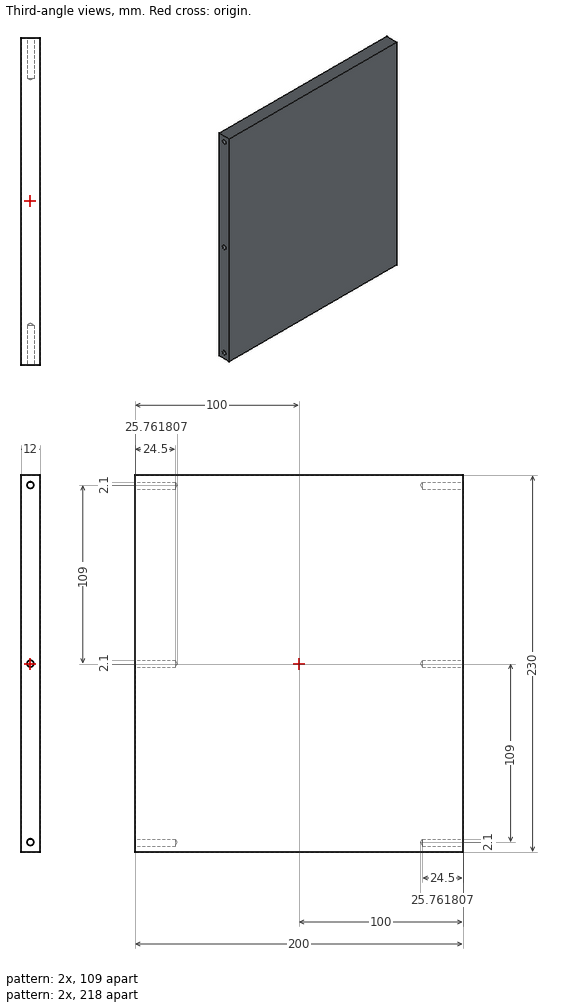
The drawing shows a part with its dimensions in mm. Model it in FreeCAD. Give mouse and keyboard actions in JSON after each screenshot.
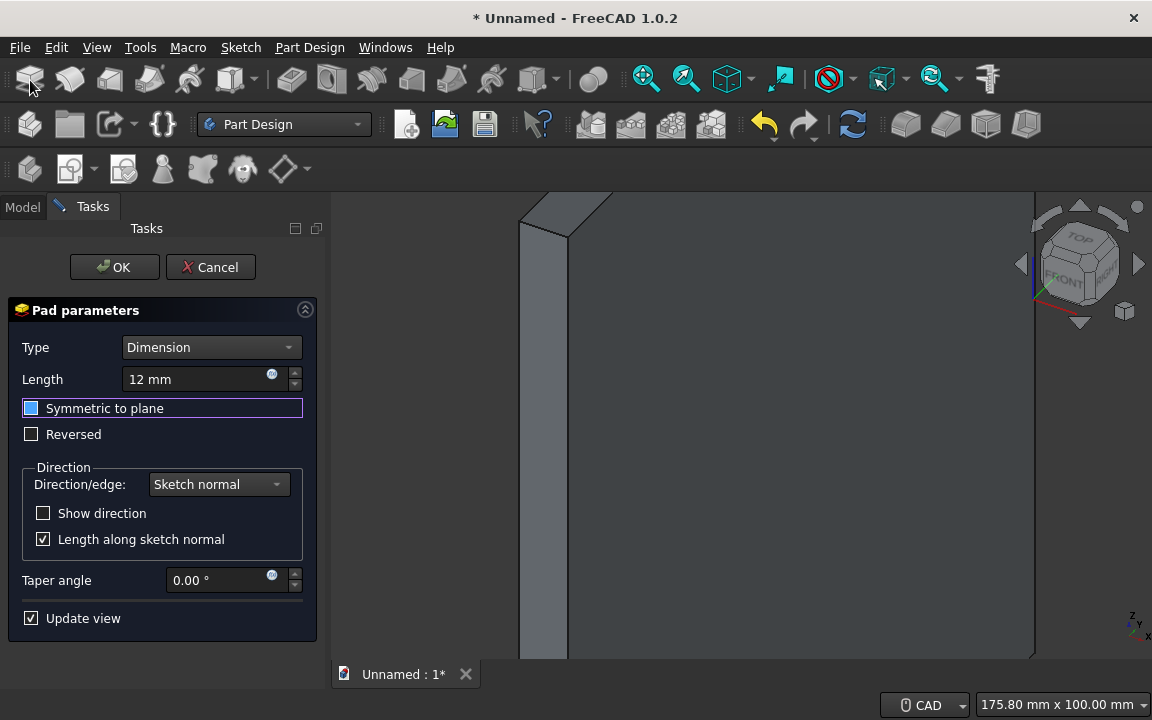
{"action": "left_click", "coordinate": [30, 408]}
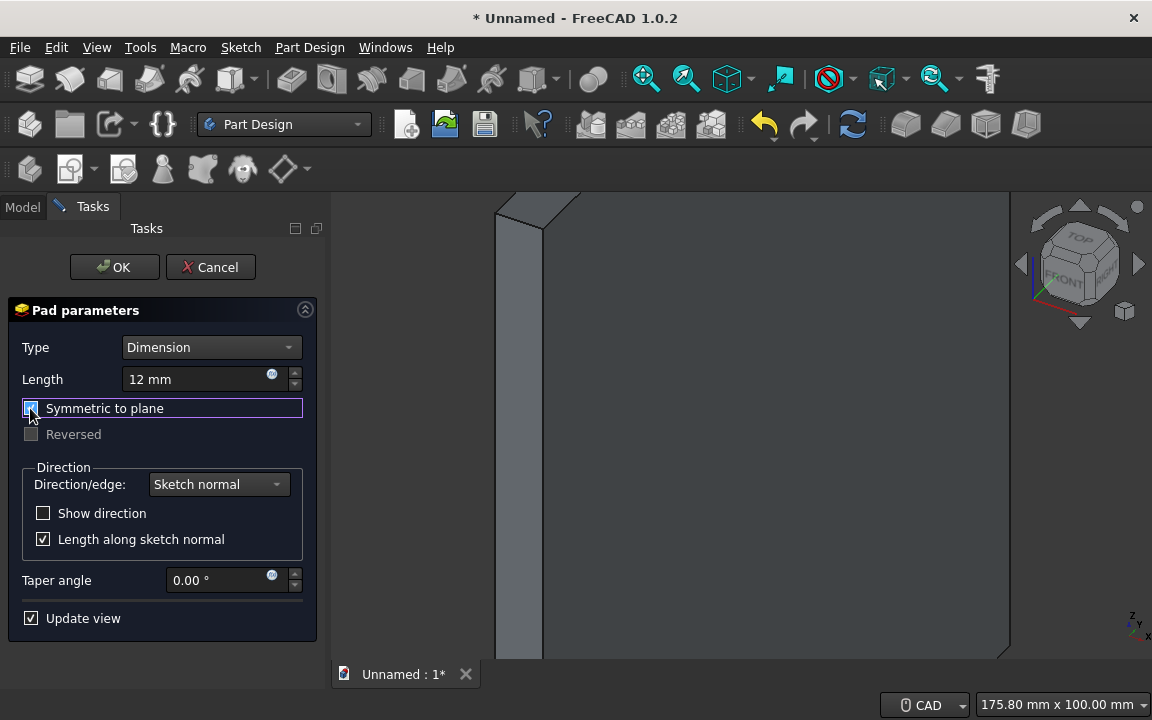
{"action": "left_click", "coordinate": [115, 267]}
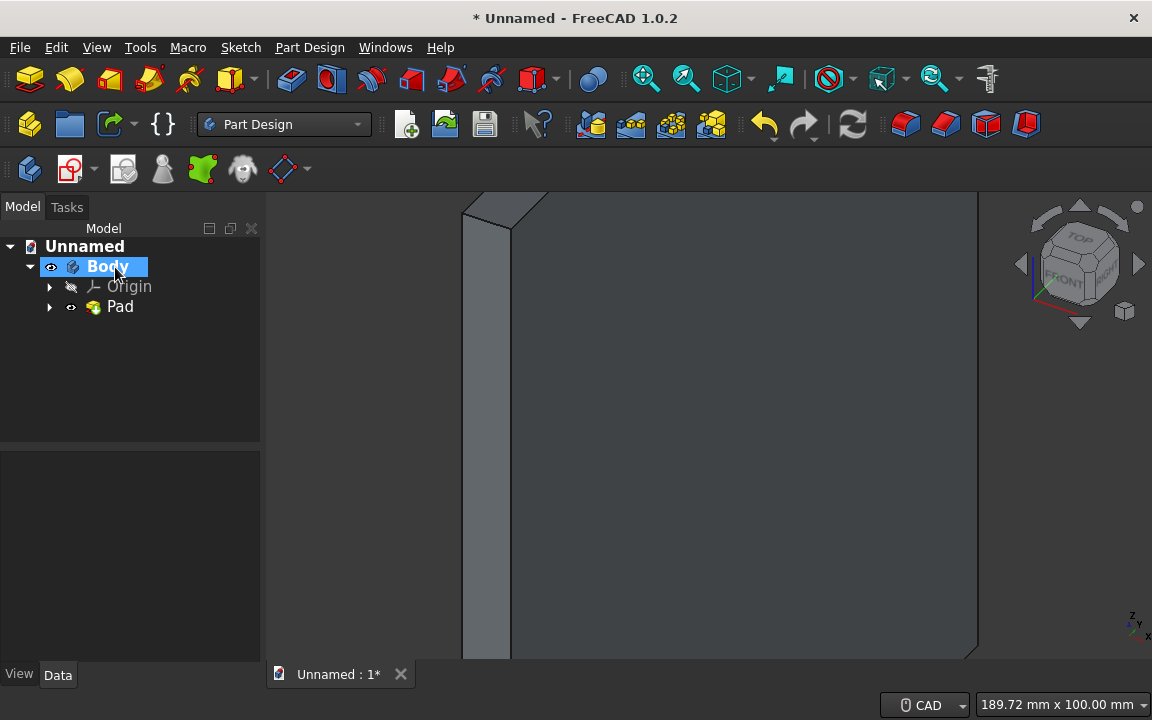
{"action": "left_click", "coordinate": [648, 80]}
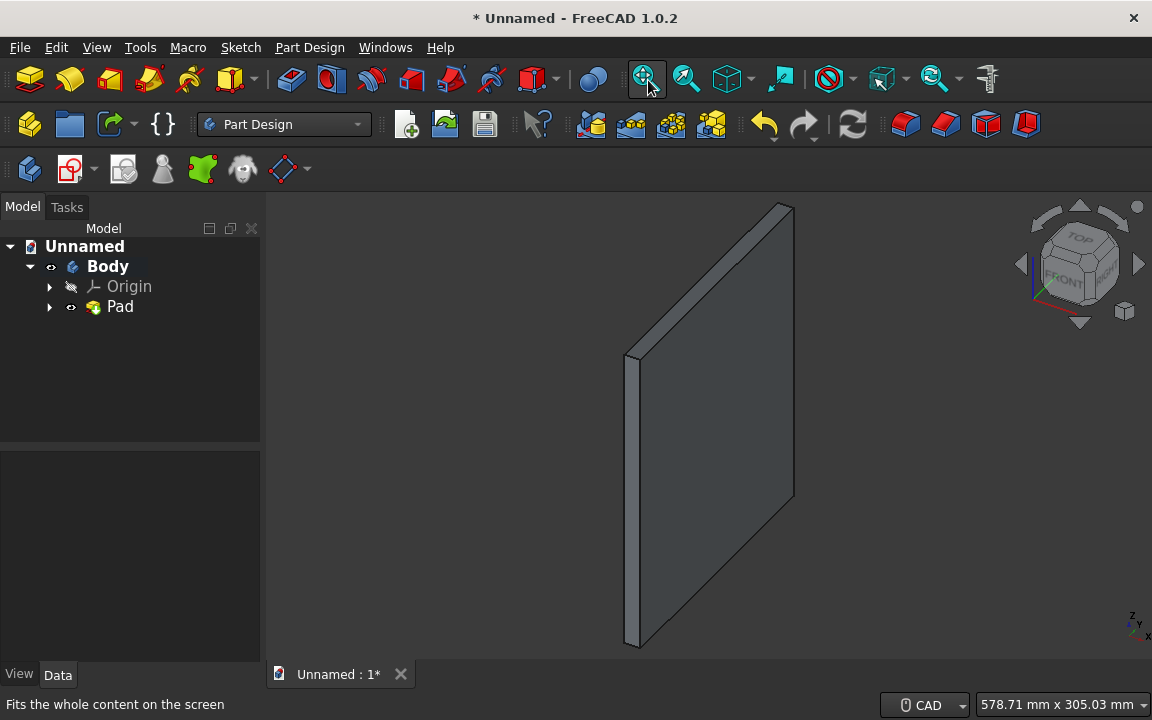
{"action": "left_click", "coordinate": [70, 170]}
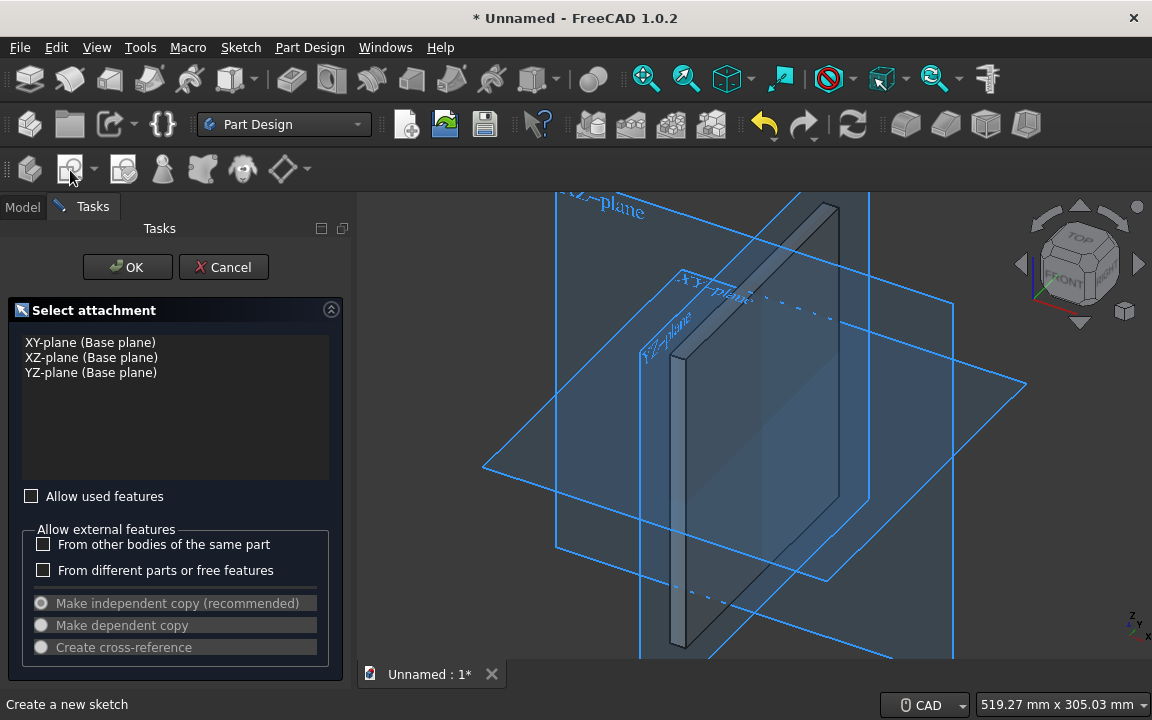
{"action": "left_click", "coordinate": [82, 372]}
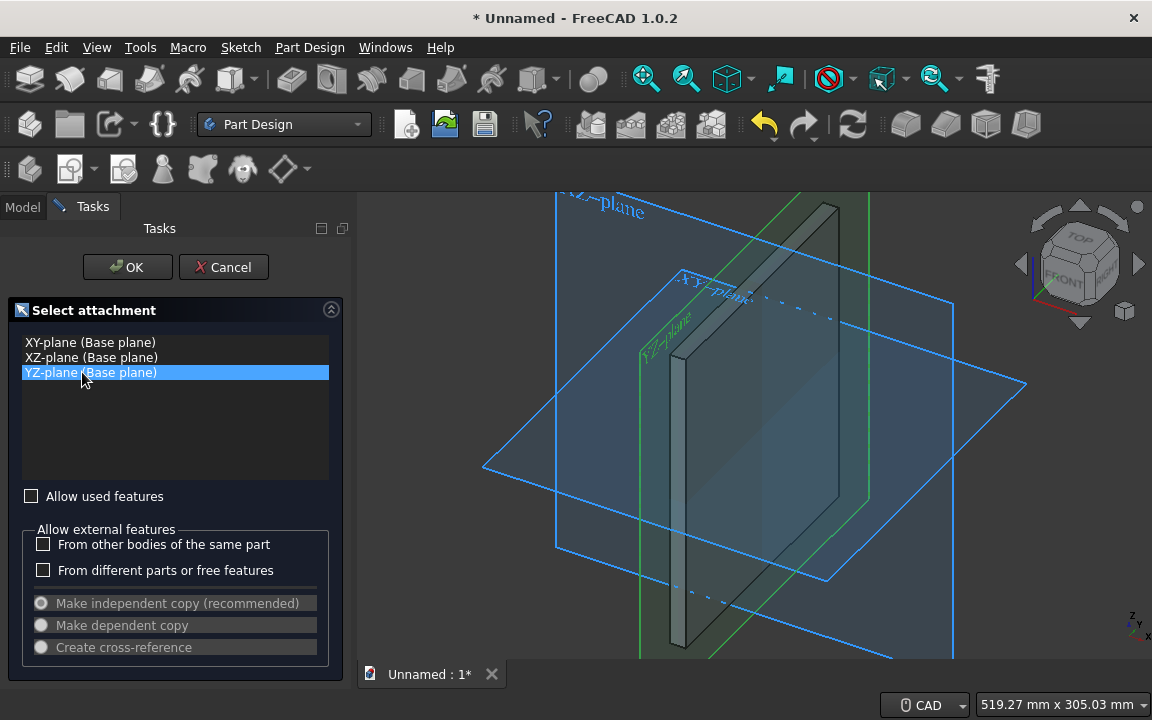
{"action": "left_click", "coordinate": [128, 267]}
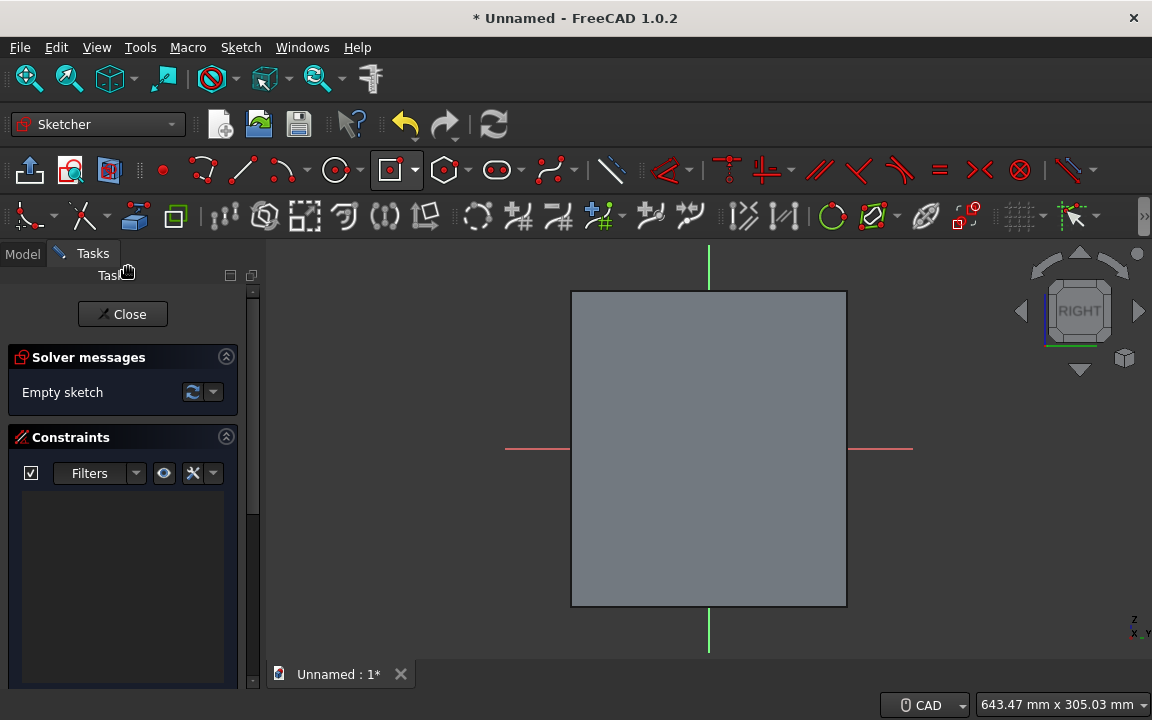
{"action": "left_click", "coordinate": [110, 170]}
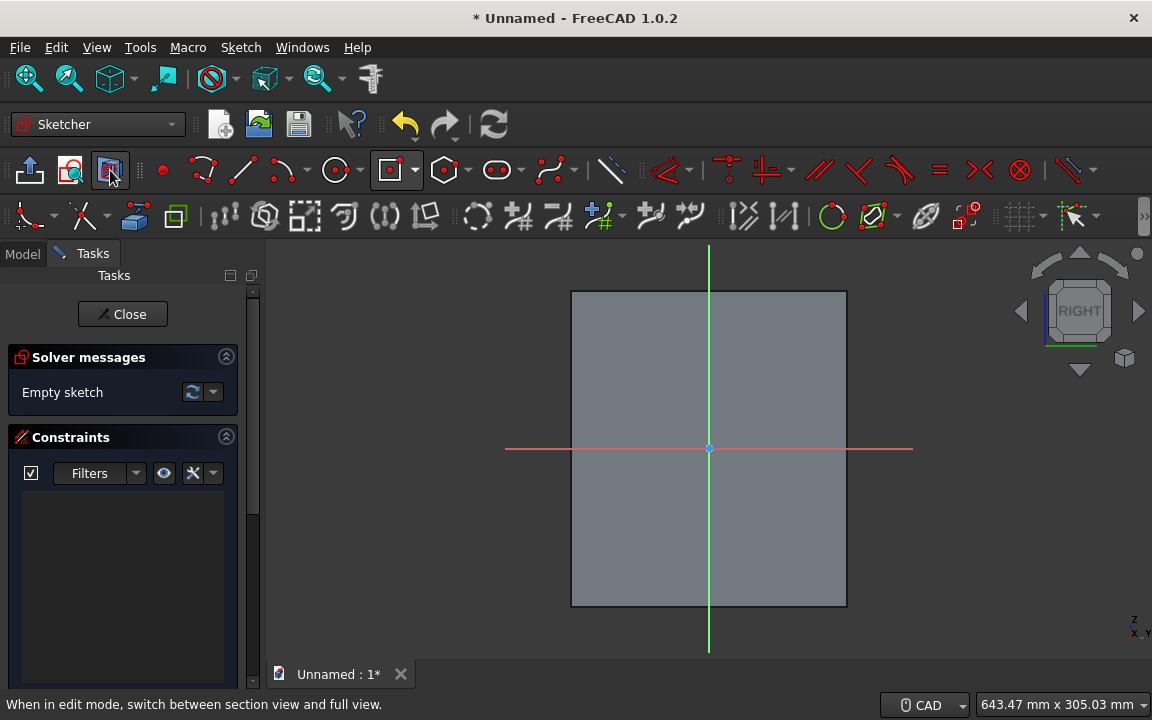
{"action": "scroll", "coordinate": [844, 616], "scroll_direction": "up", "scroll_amount": 11}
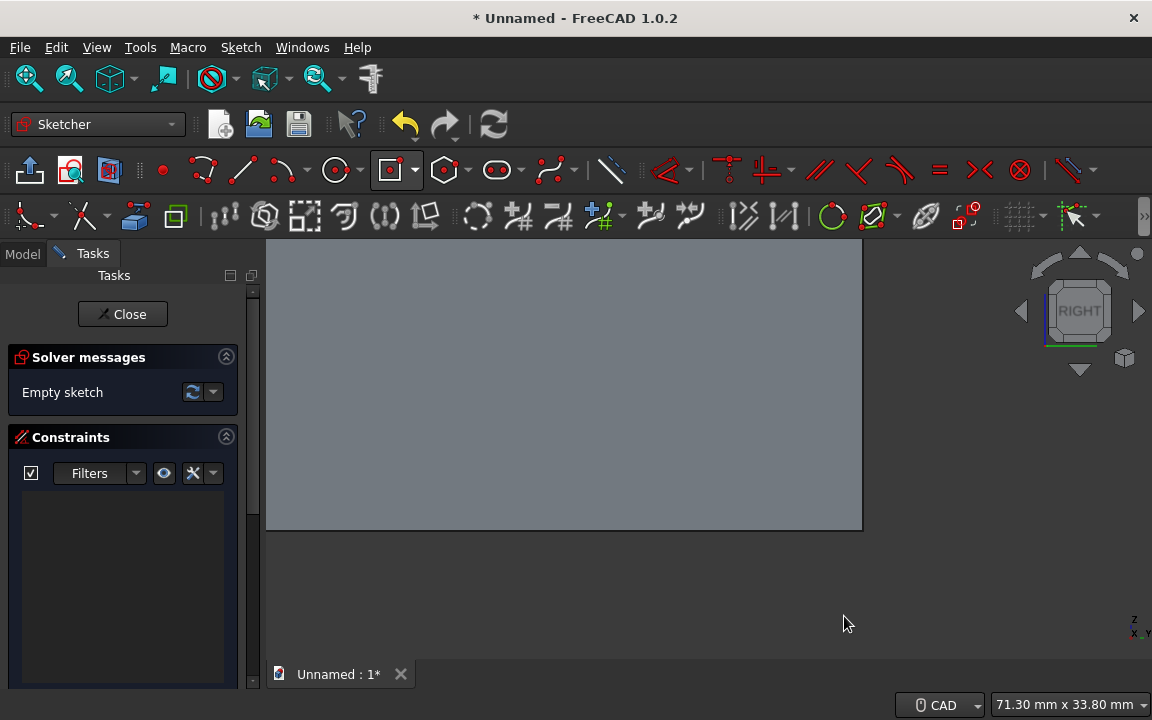
{"action": "left_click", "coordinate": [204, 170]}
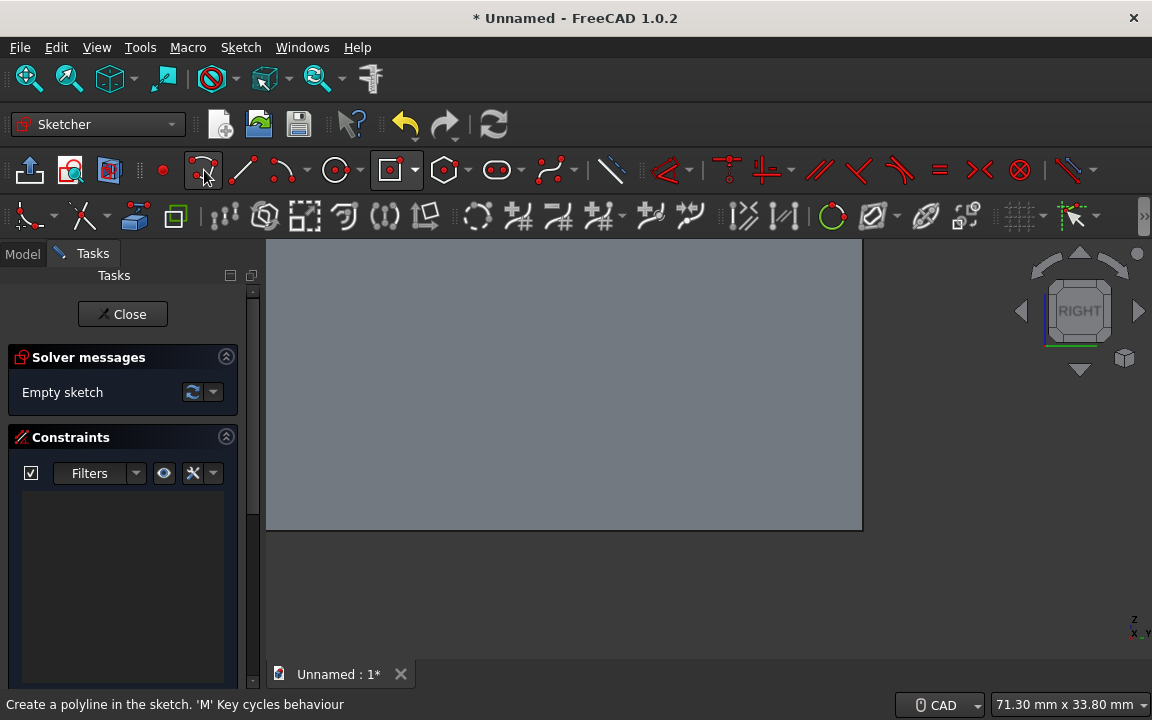
{"action": "left_click", "coordinate": [559, 430]}
{"action": "left_click", "coordinate": [543, 456]}
{"action": "left_click", "coordinate": [863, 456]}
{"action": "left_click", "coordinate": [863, 430]}
{"action": "left_click", "coordinate": [559, 431]}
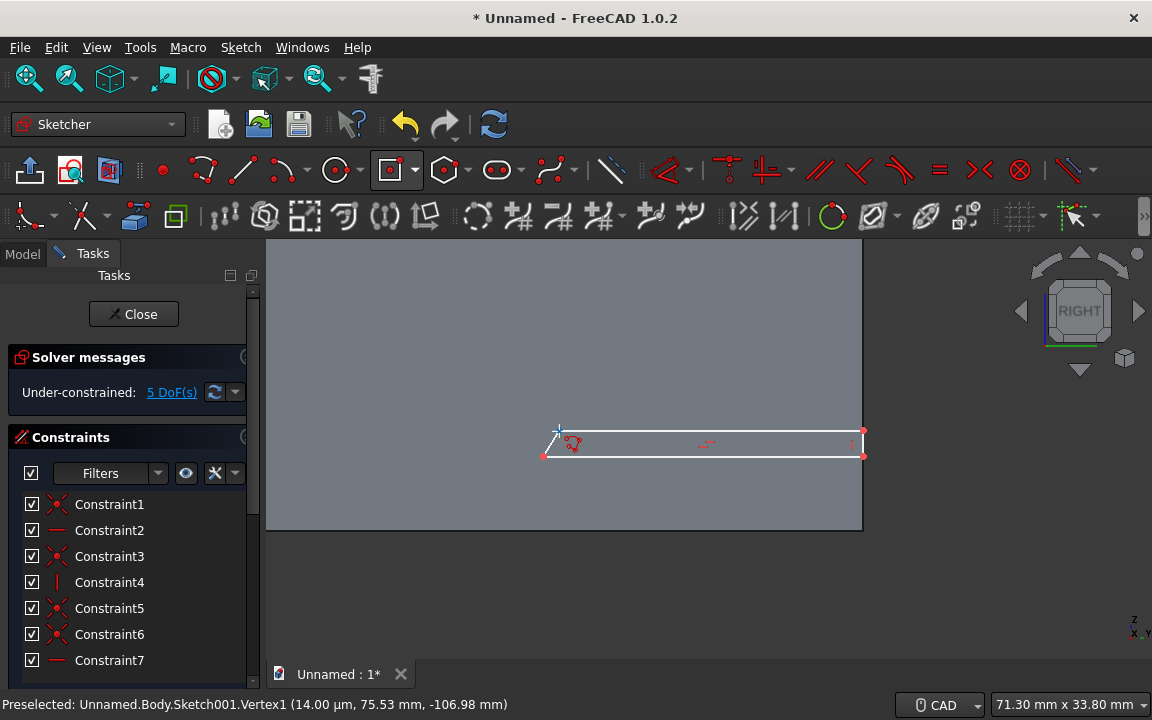
{"action": "left_click", "coordinate": [244, 170]}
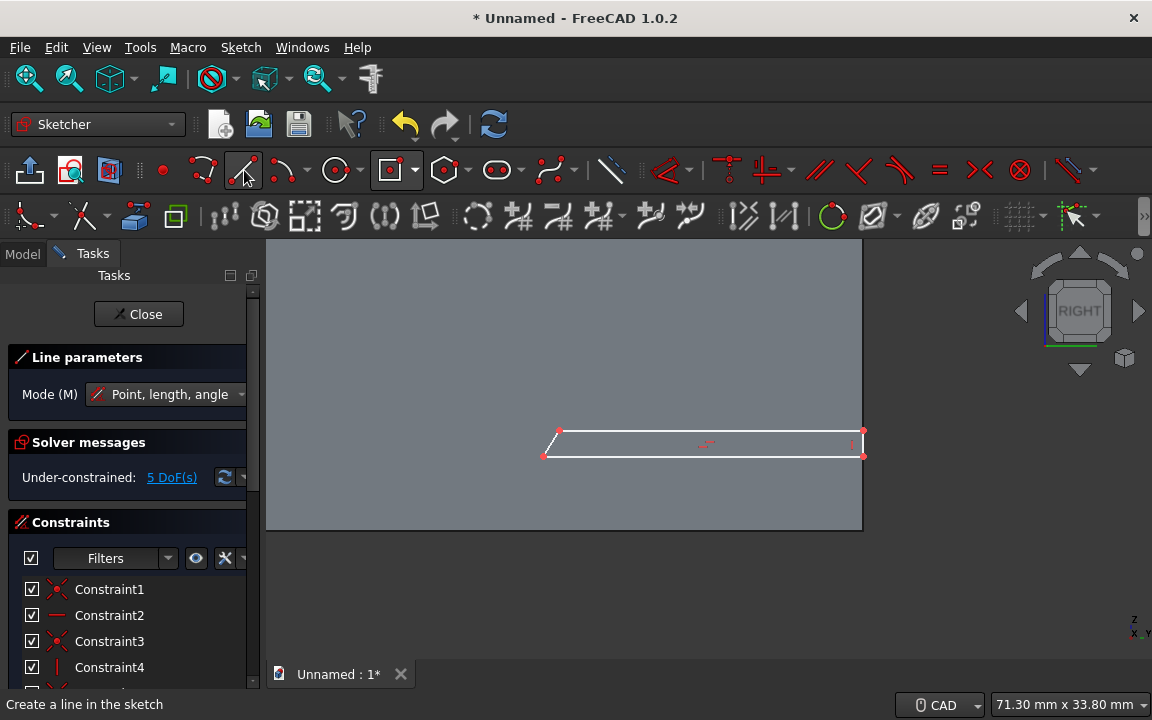
{"action": "left_click", "coordinate": [511, 456]}
{"action": "left_click", "coordinate": [415, 456]}
{"action": "key", "text": "Escape"}